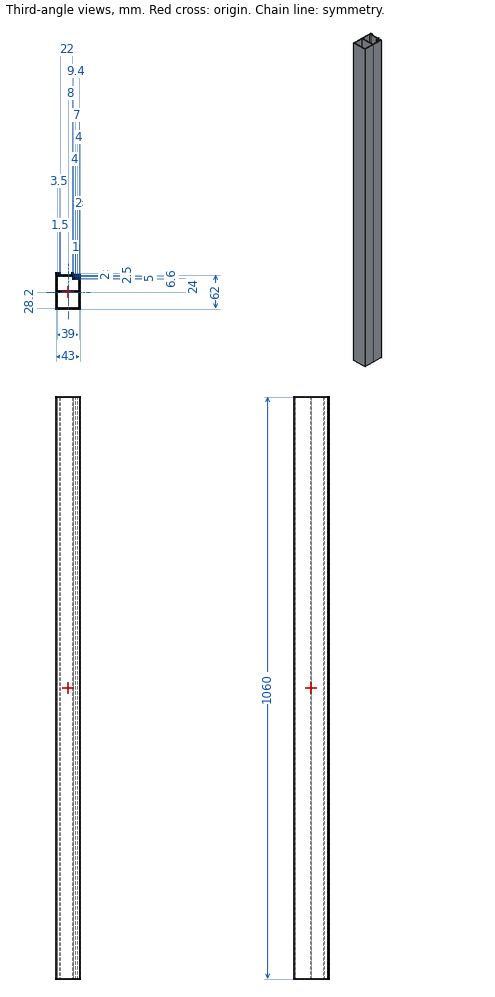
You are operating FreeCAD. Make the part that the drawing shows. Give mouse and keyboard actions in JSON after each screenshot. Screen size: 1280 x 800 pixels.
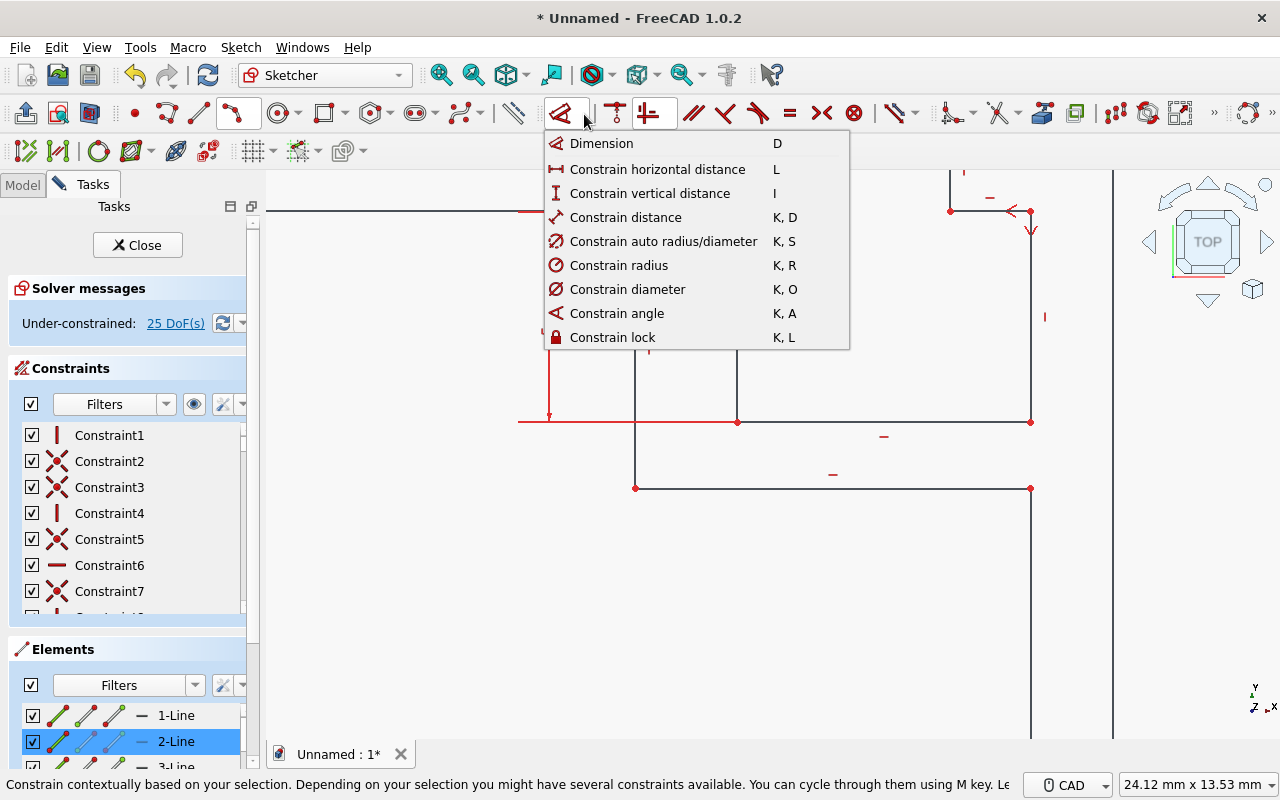
{"action": "left_click", "coordinate": [697, 169]}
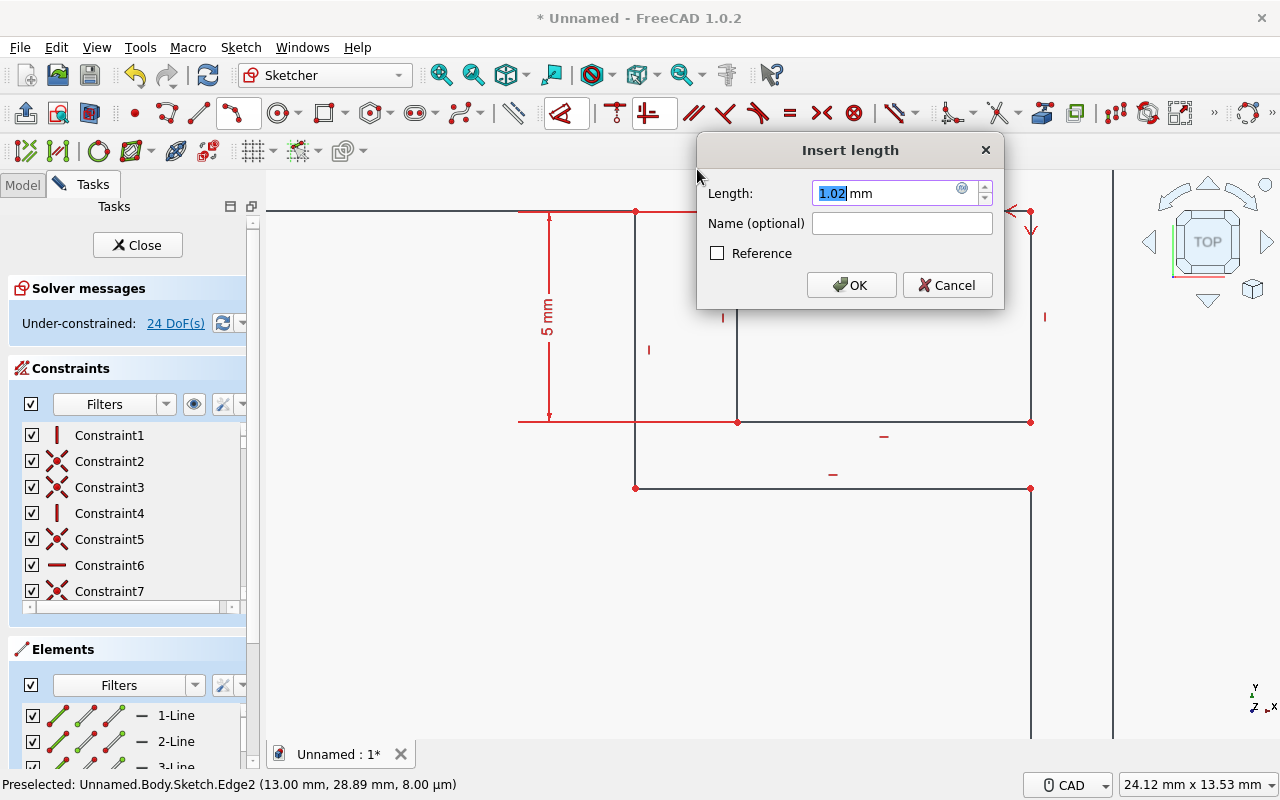
{"action": "type", "text": "1"}
{"action": "key", "text": "Return"}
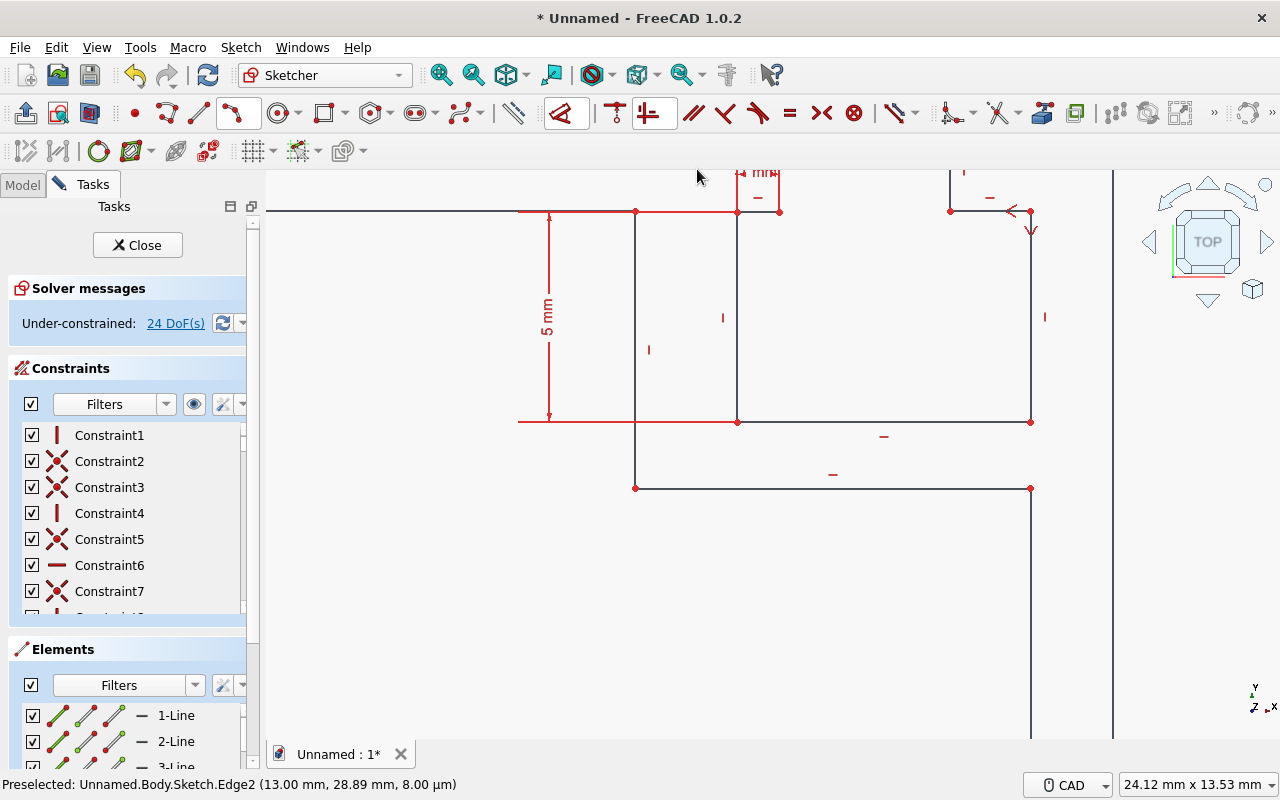
{"action": "scroll", "coordinate": [781, 311], "scroll_direction": "down", "scroll_amount": 10}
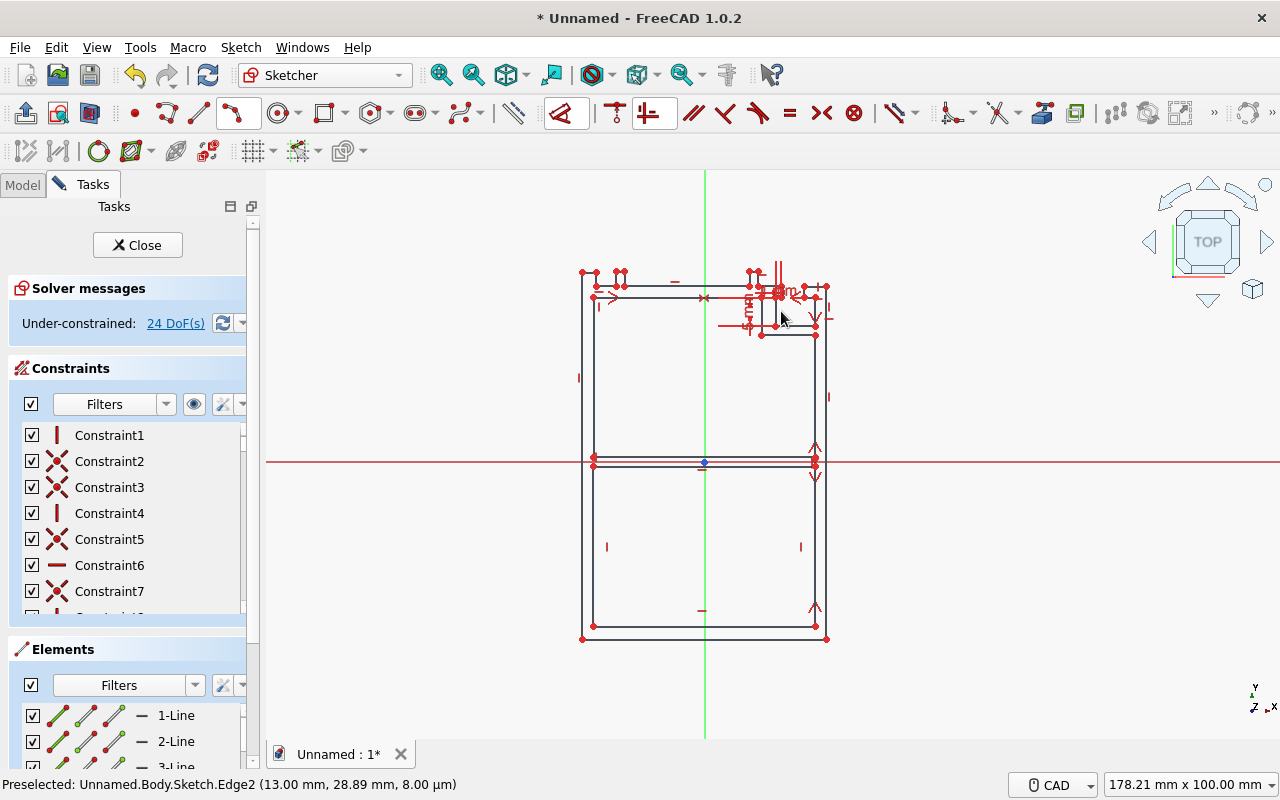
{"action": "scroll", "coordinate": [781, 294], "scroll_direction": "up", "scroll_amount": 7}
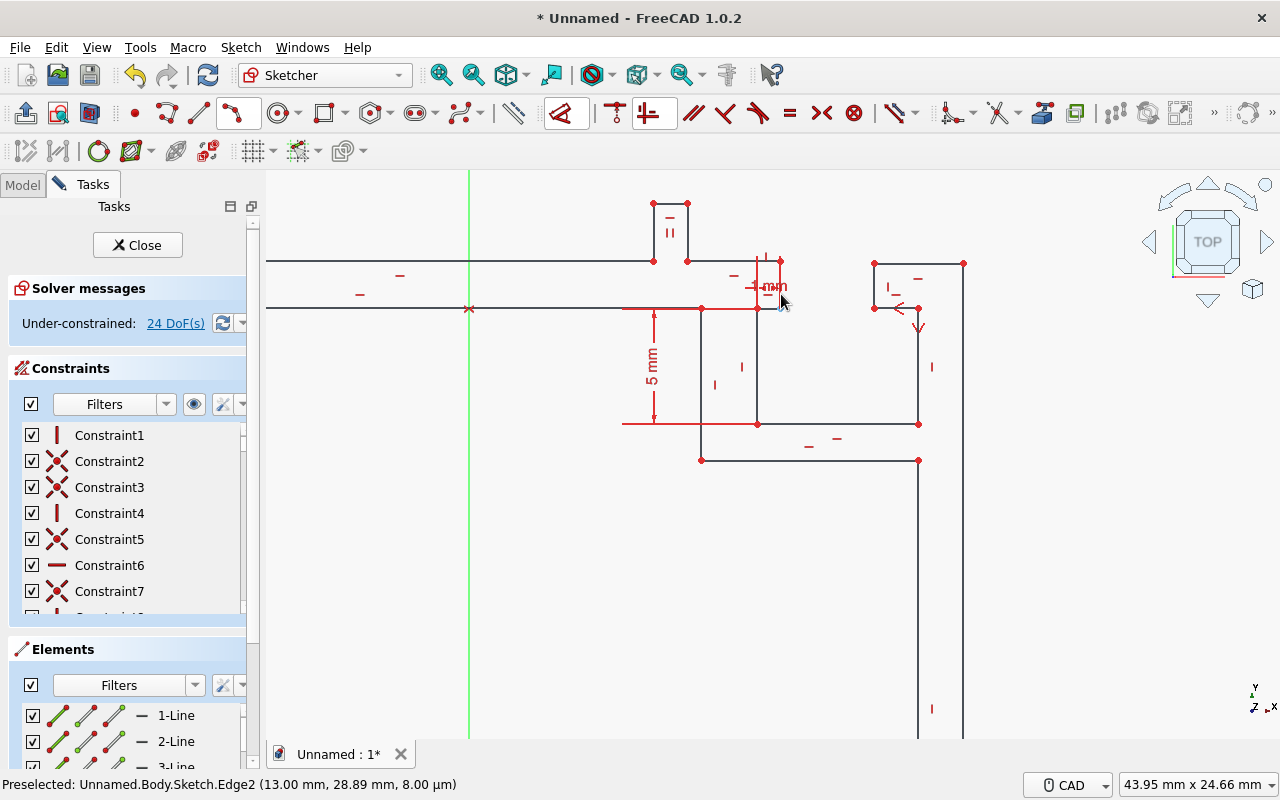
{"action": "left_click", "coordinate": [780, 275]}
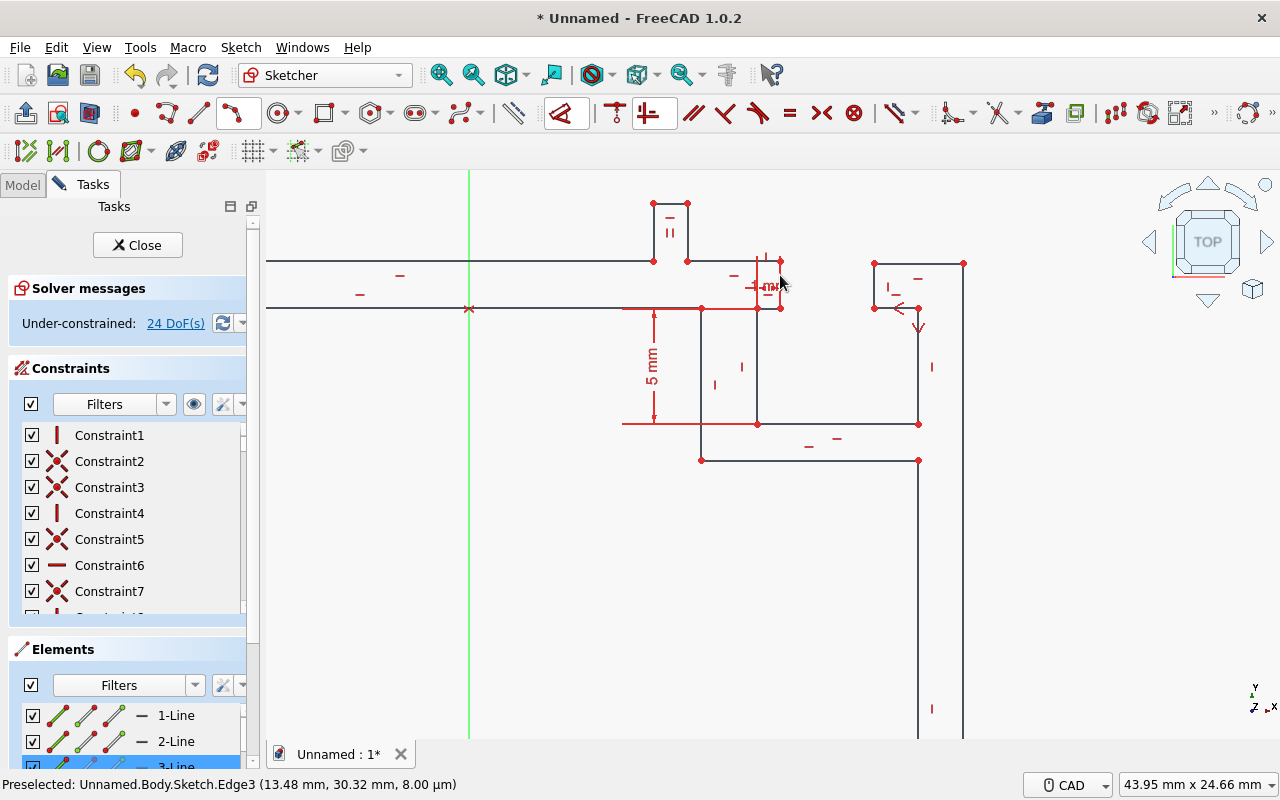
{"action": "key", "text": "i"}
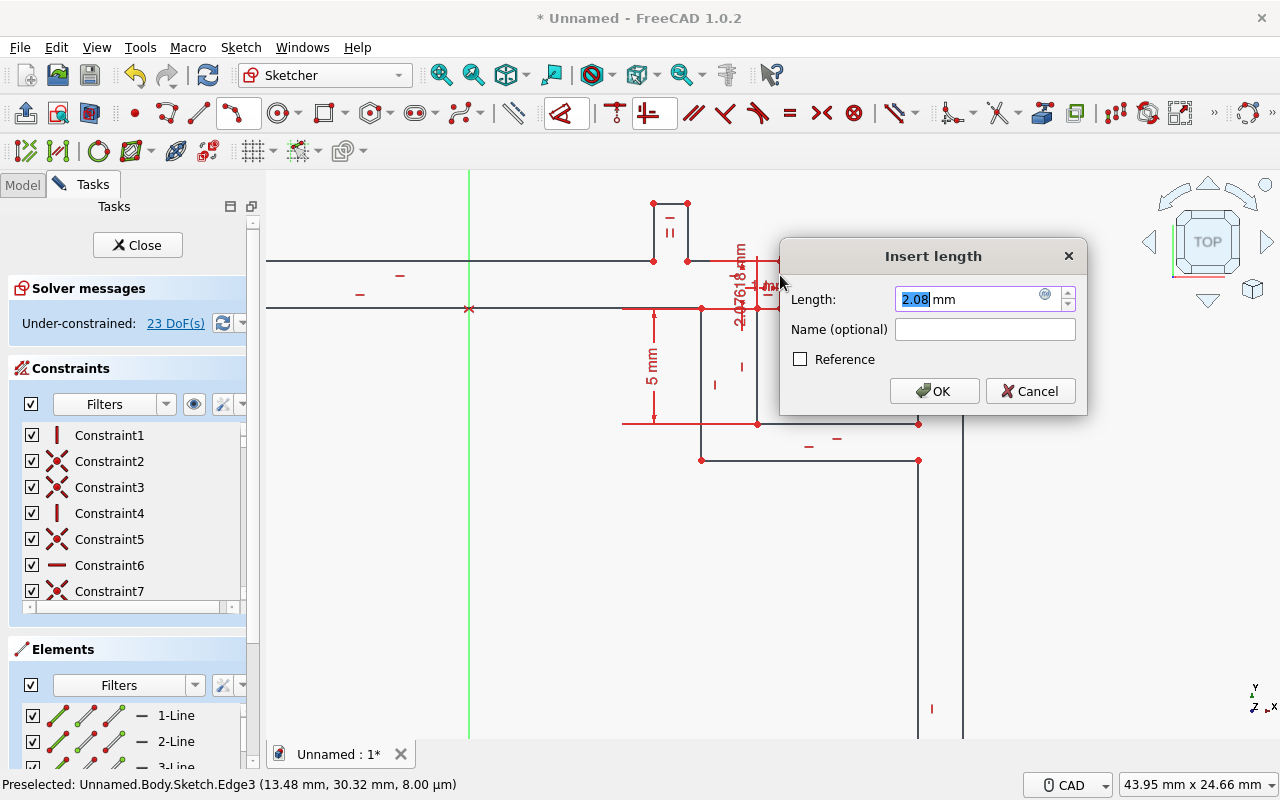
{"action": "type", "text": "2"}
{"action": "key", "text": "Return"}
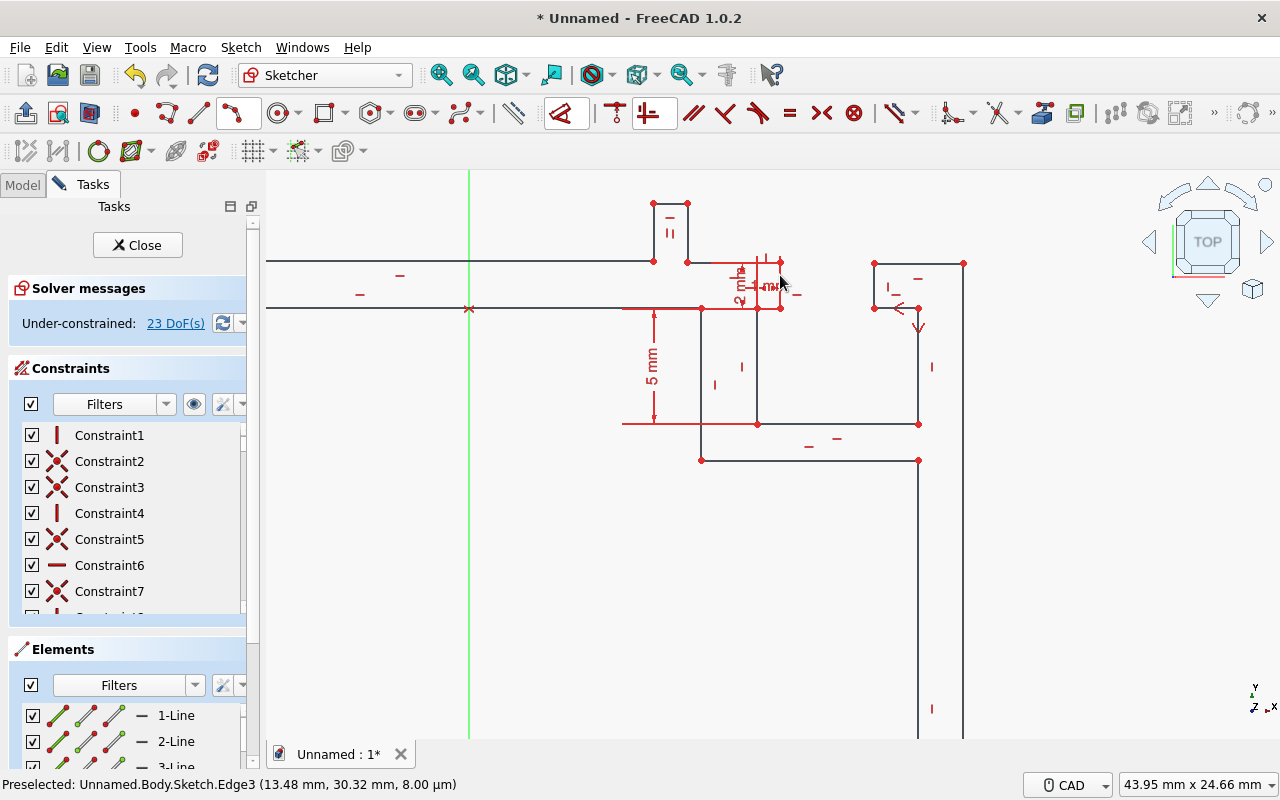
{"action": "left_click", "coordinate": [753, 263]}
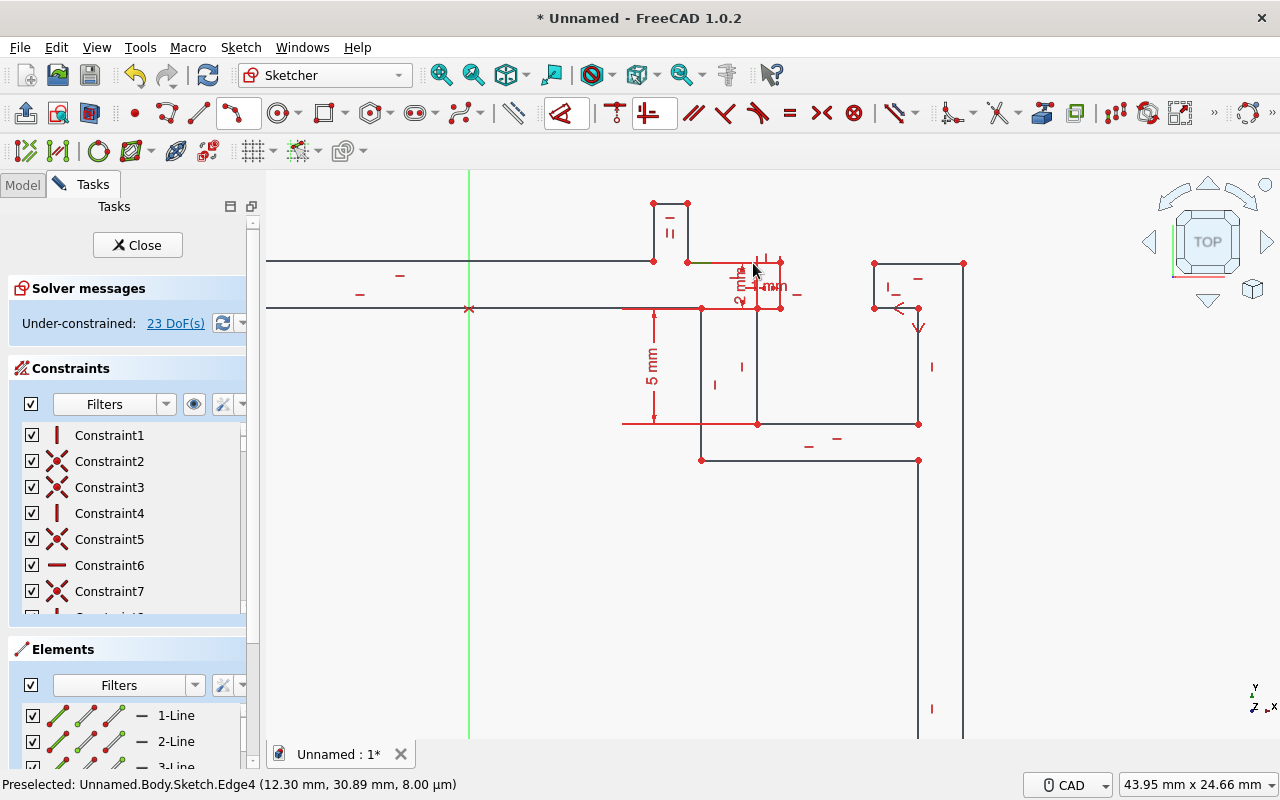
{"action": "key", "text": "l"}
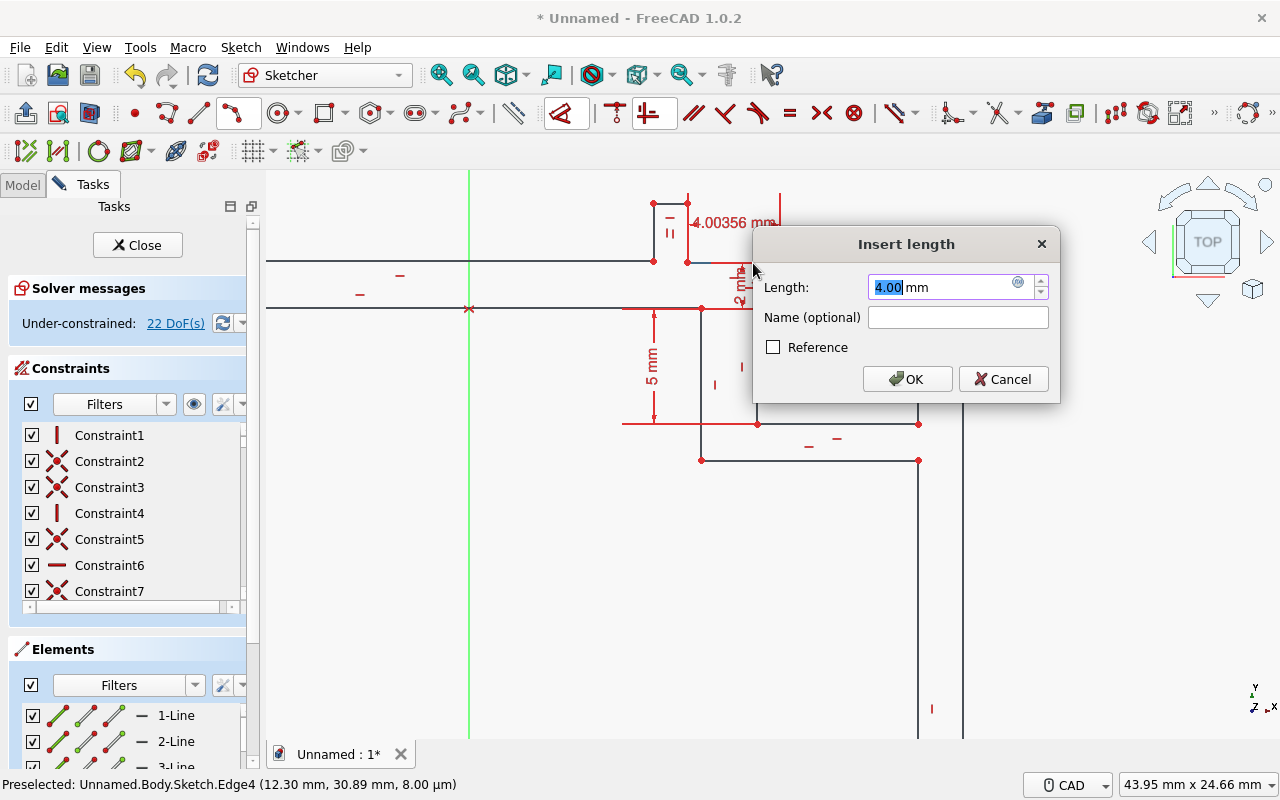
{"action": "type", "text": "4"}
{"action": "key", "text": "Return"}